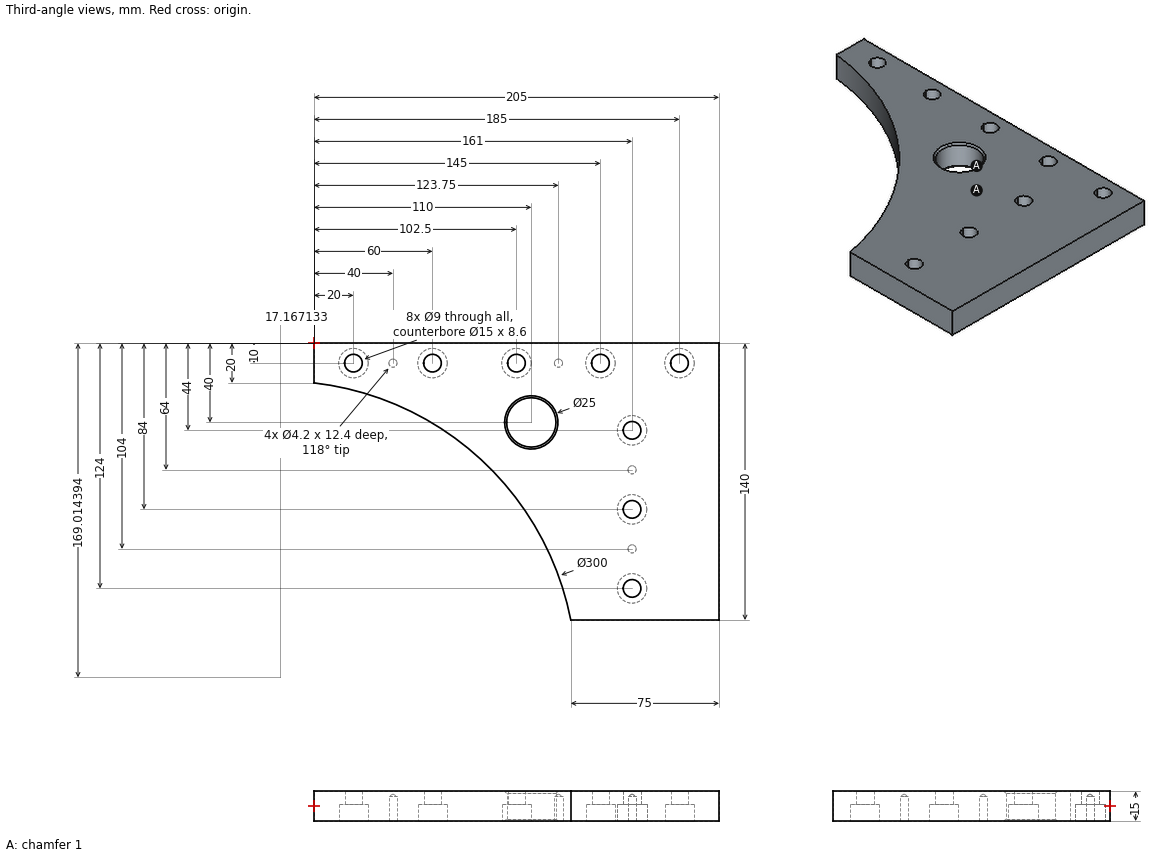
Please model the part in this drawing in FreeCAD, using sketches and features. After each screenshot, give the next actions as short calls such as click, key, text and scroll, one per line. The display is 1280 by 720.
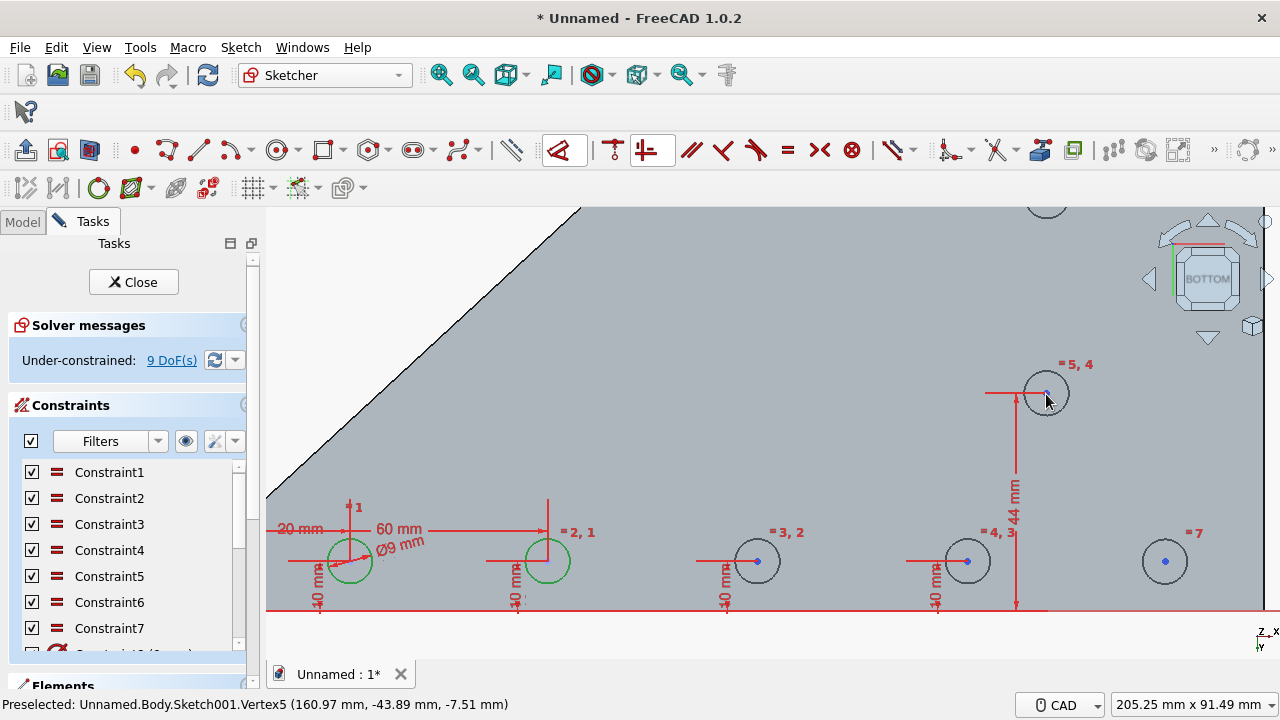
scroll(692, 547, down, 4)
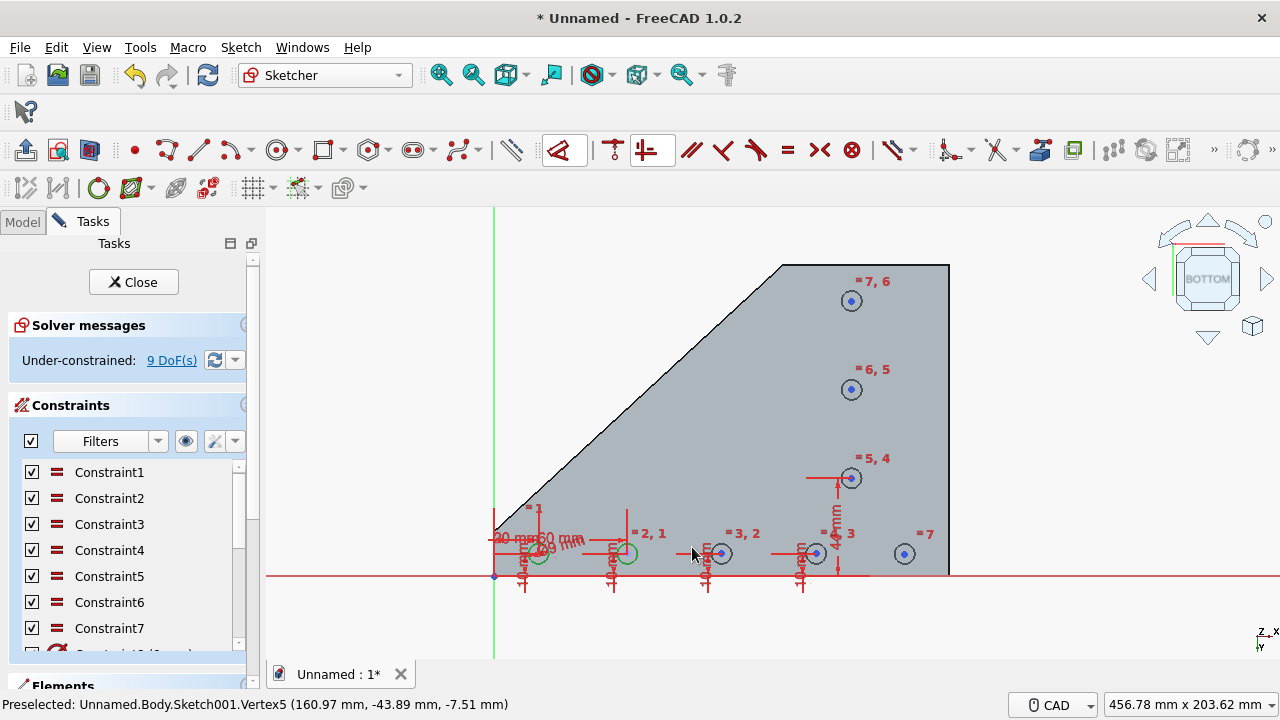
click(852, 390)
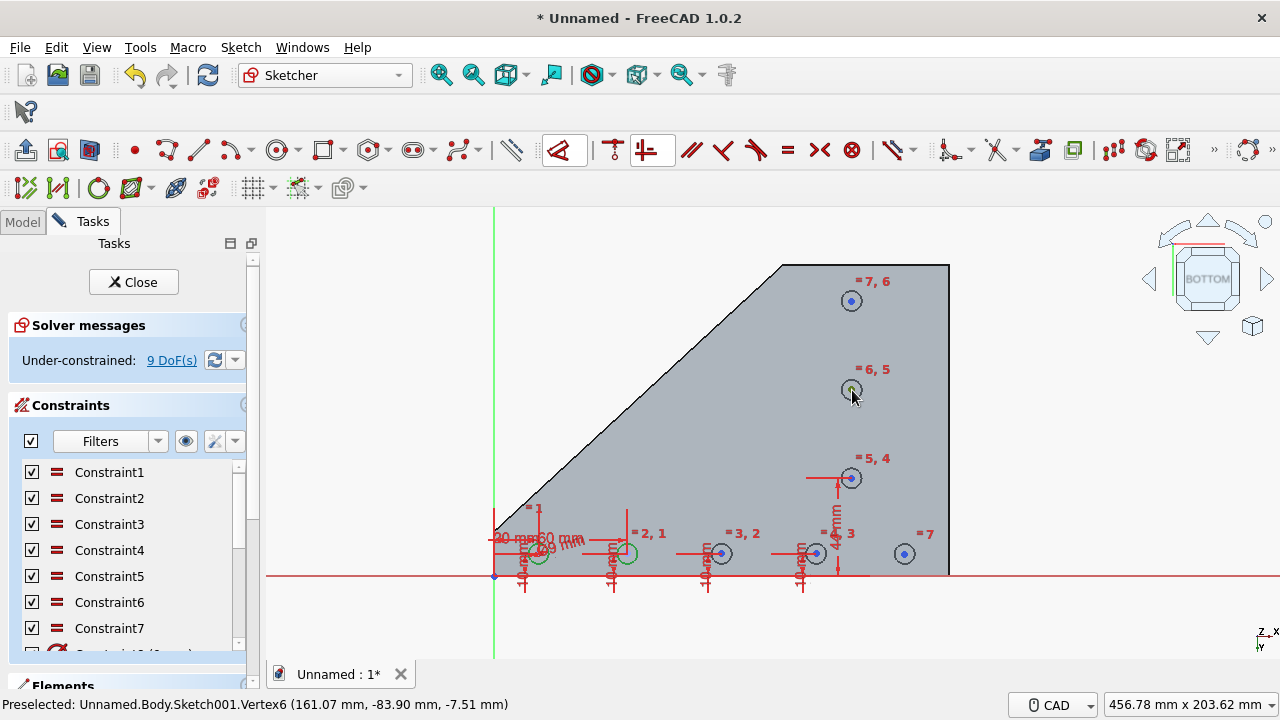
key(i)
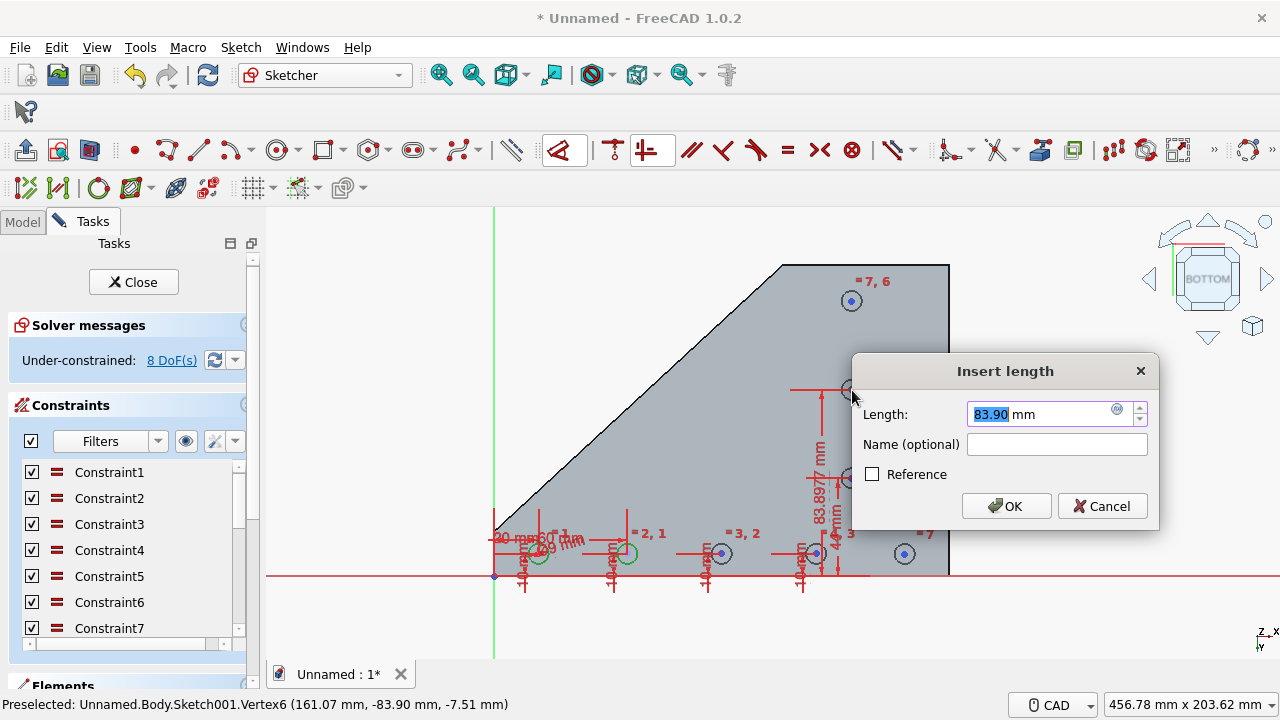
text(84)
key(Return)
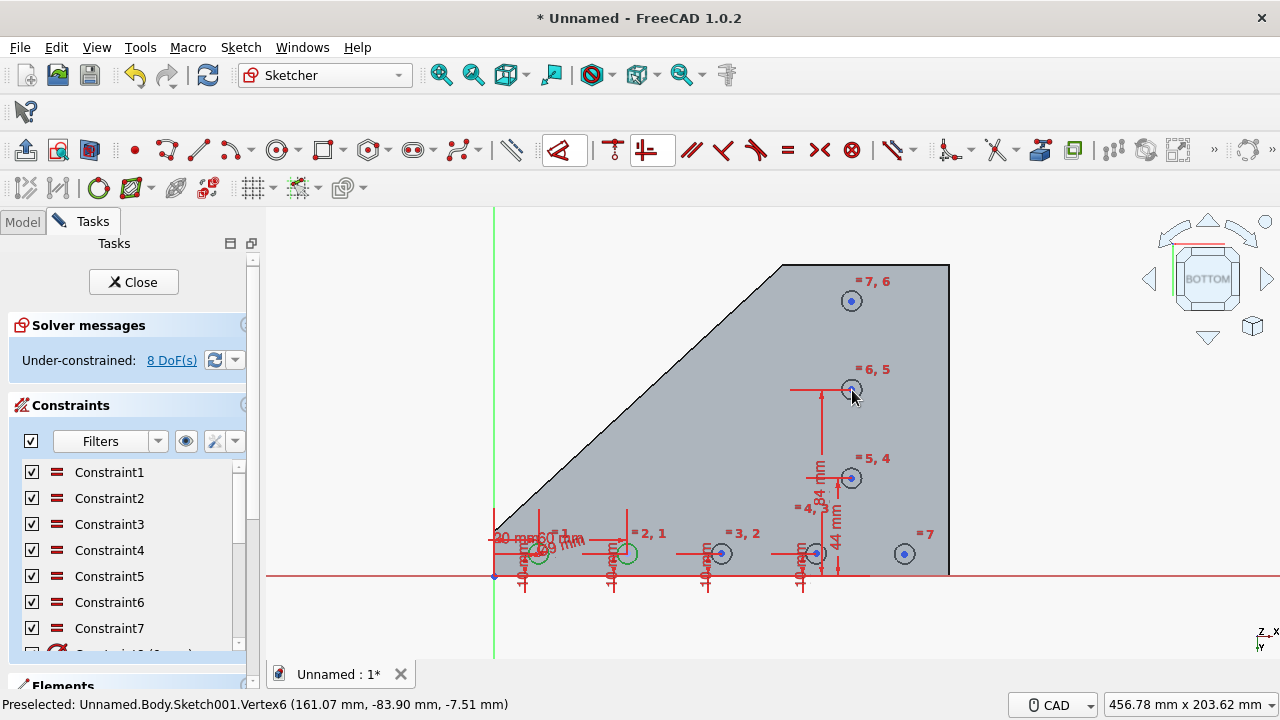
scroll(905, 554, up, 3)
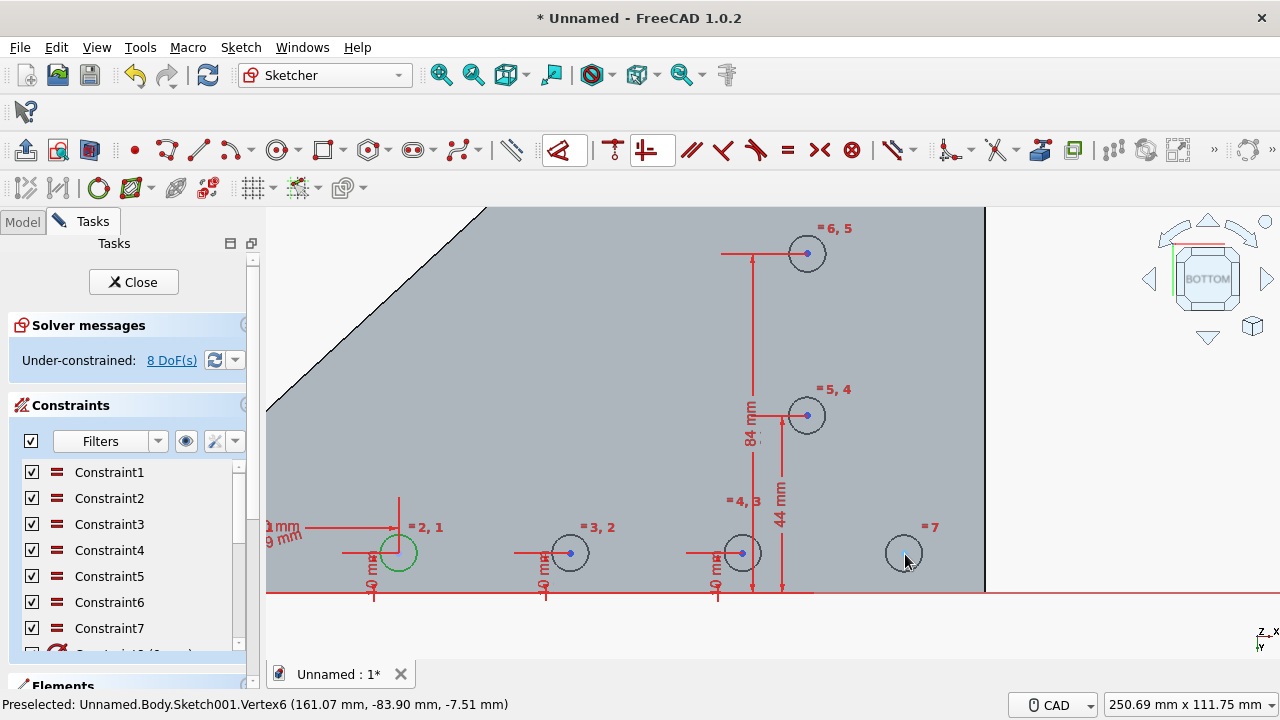
click(904, 553)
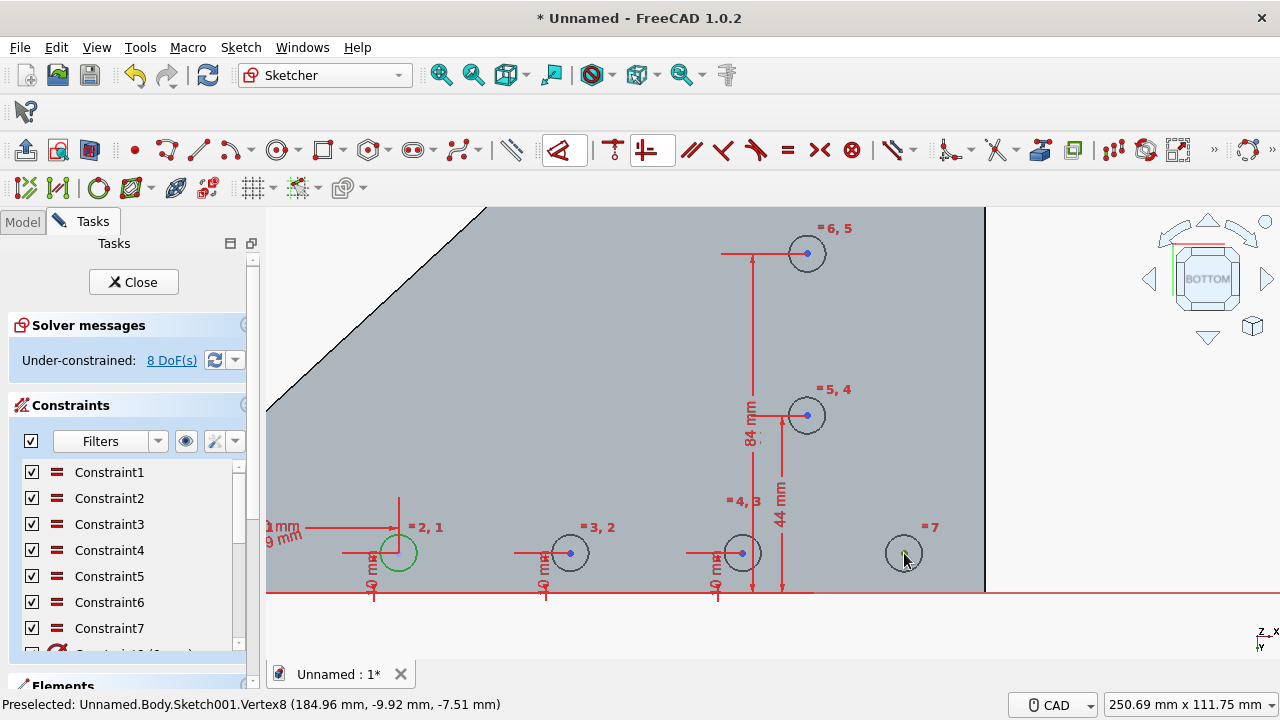
click(582, 150)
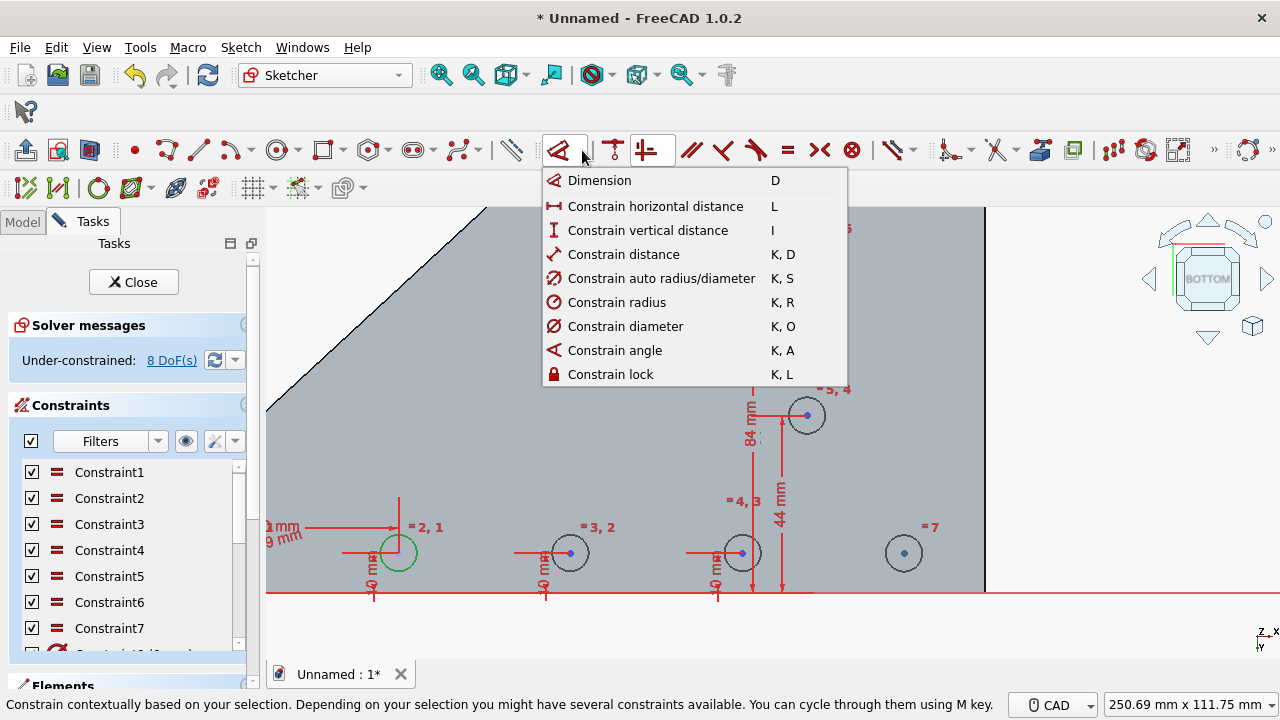
click(695, 230)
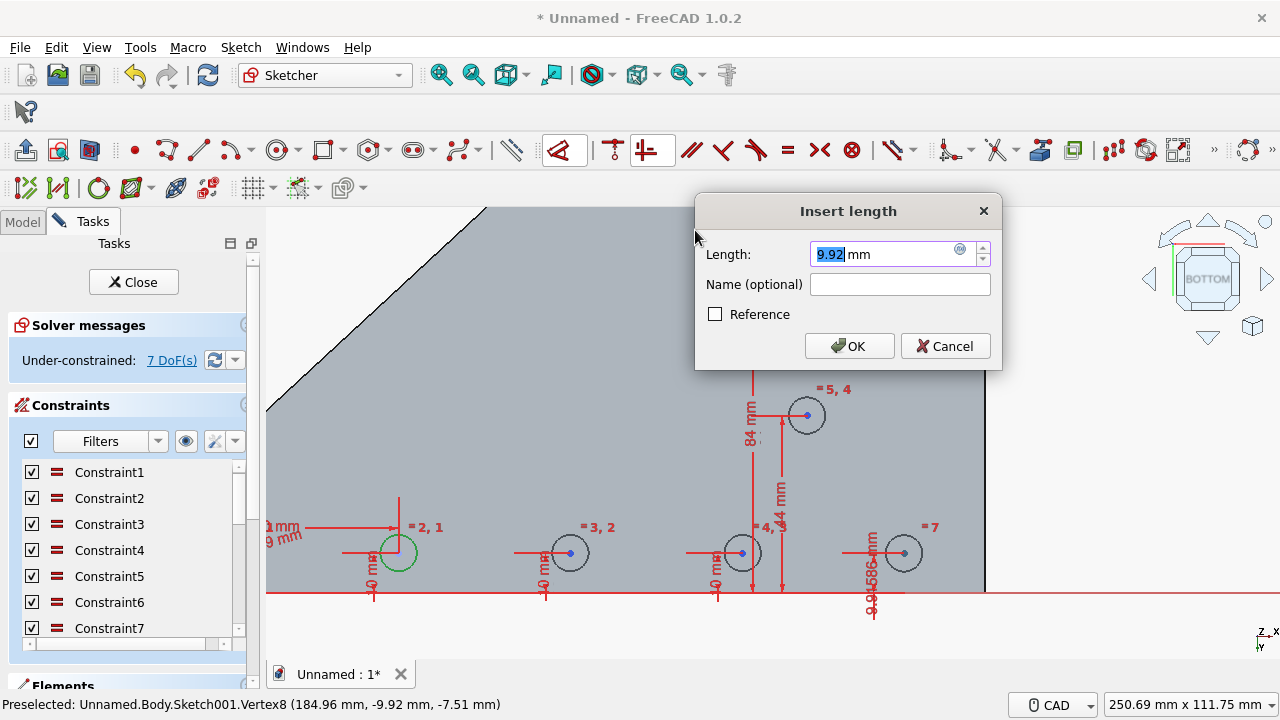
text(10)
key(Return)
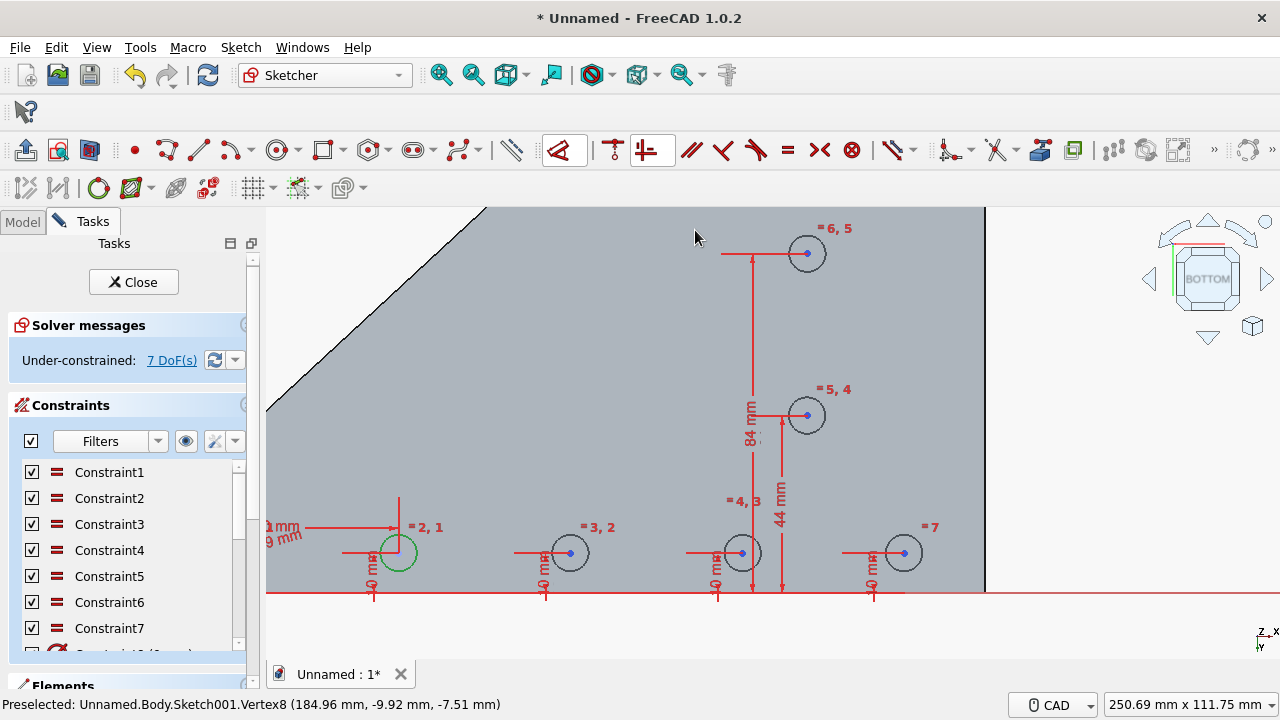
click(743, 553)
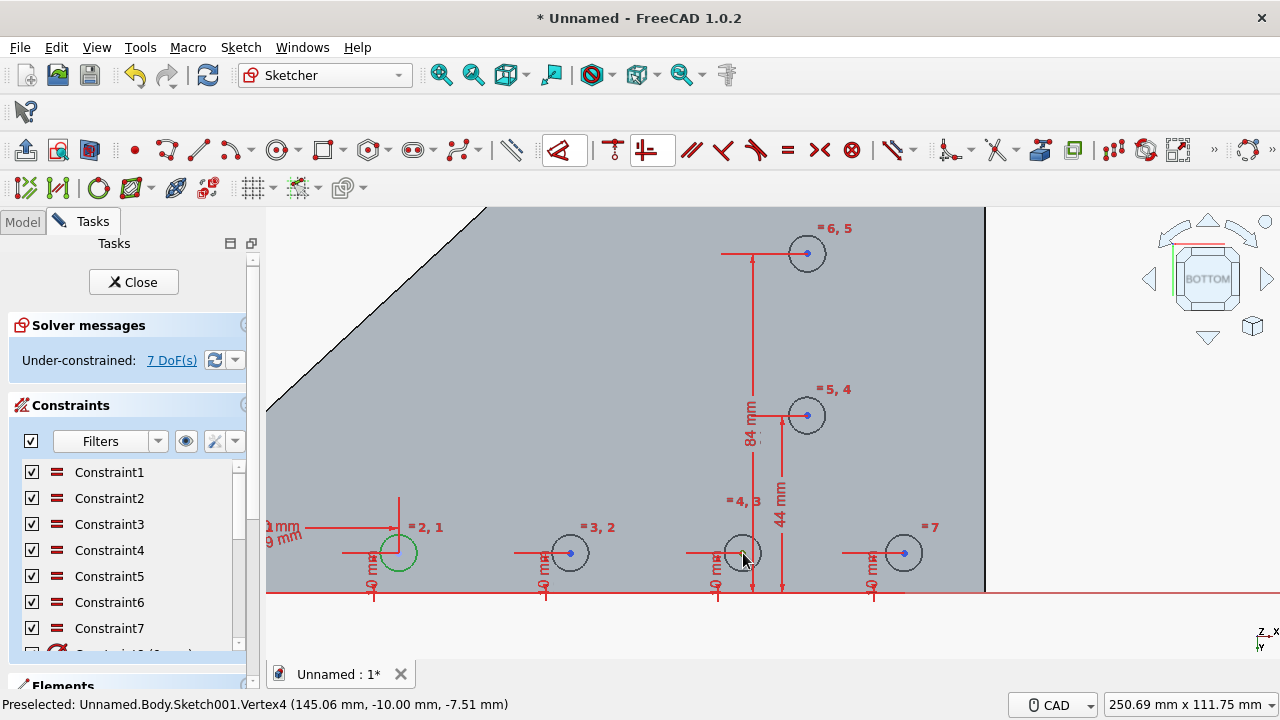
click(582, 150)